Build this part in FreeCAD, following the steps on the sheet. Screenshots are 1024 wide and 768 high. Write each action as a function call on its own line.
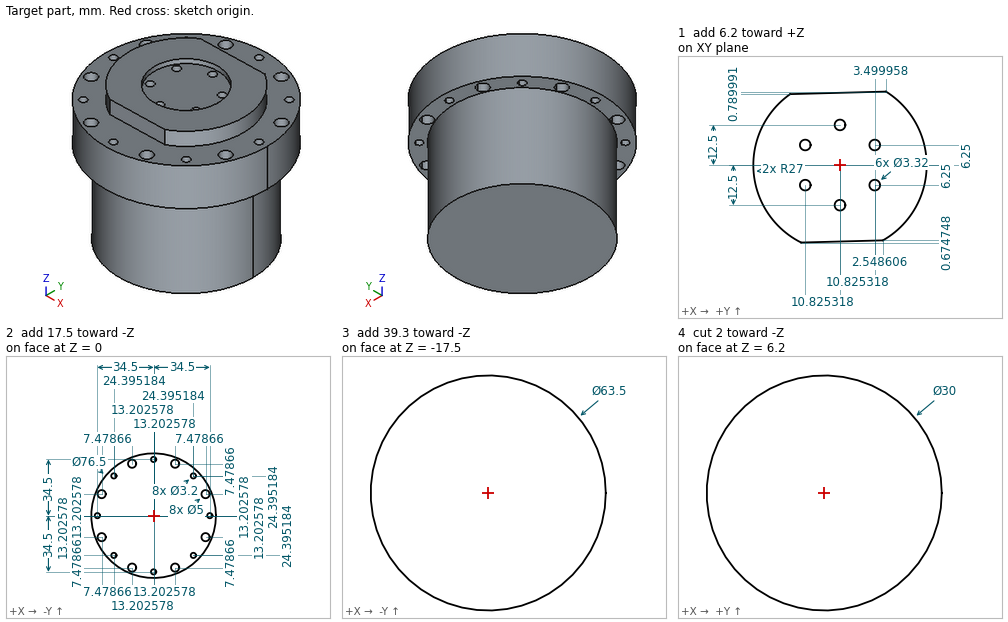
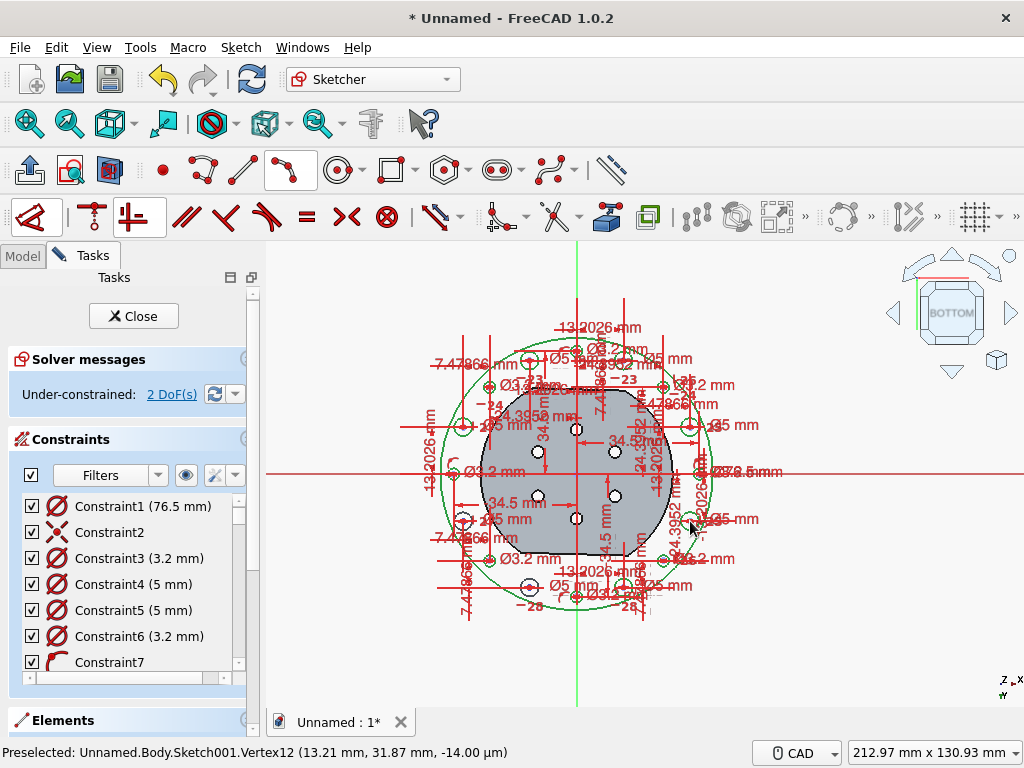
click(463, 521)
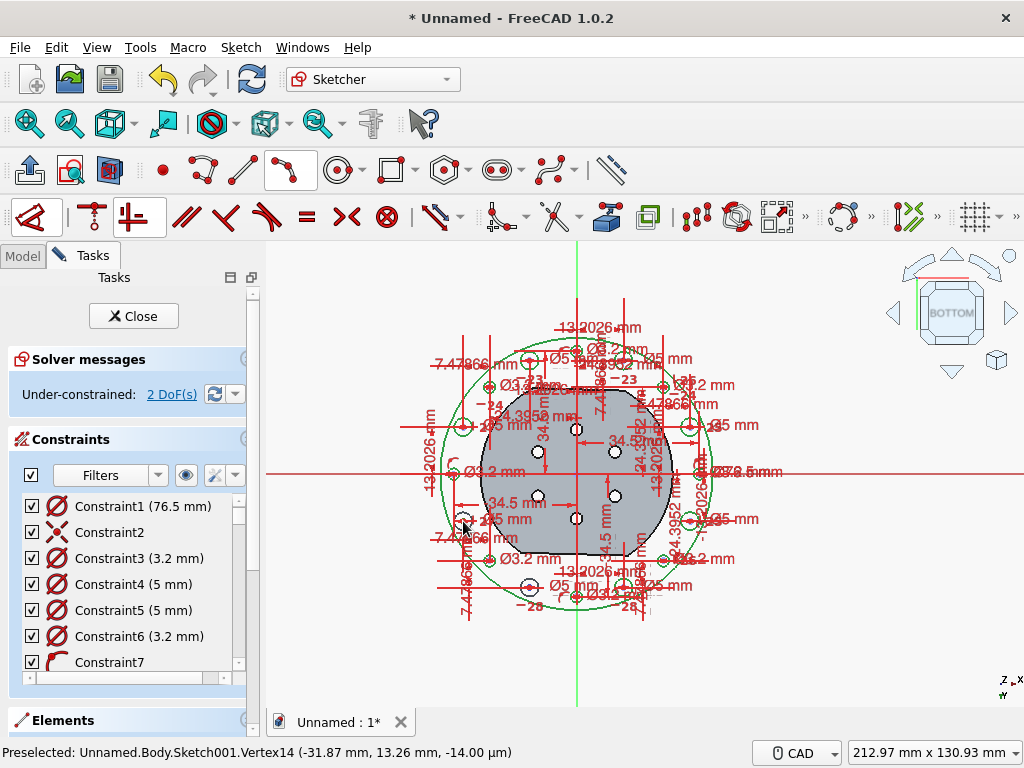
click(56, 218)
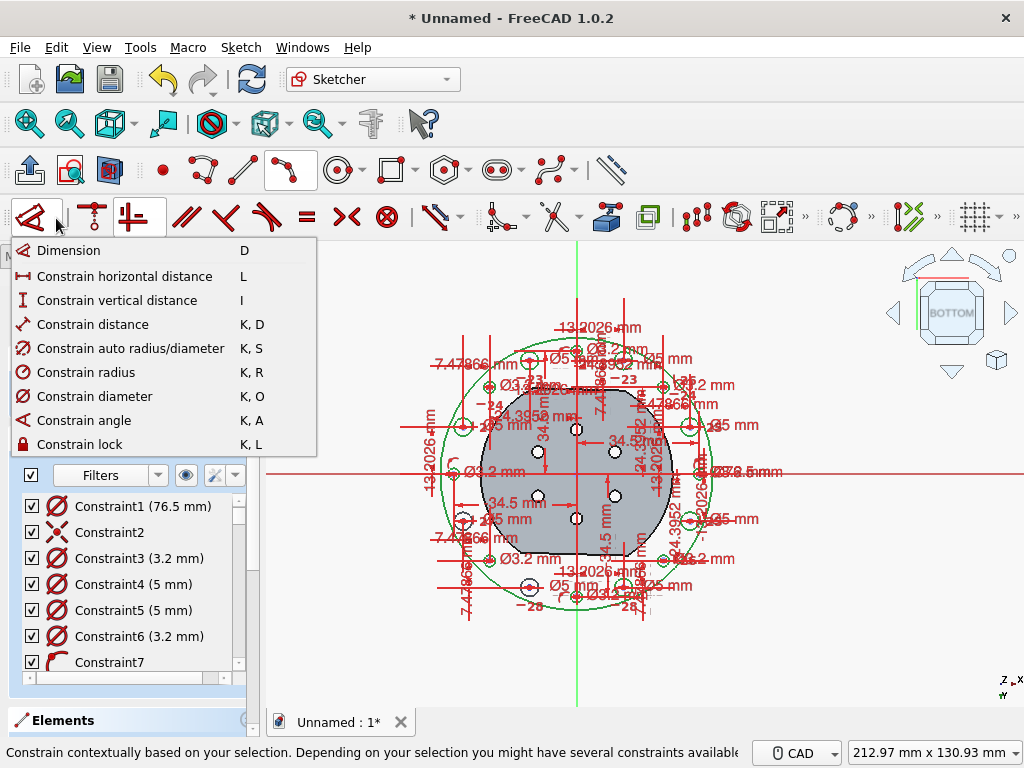
click(164, 300)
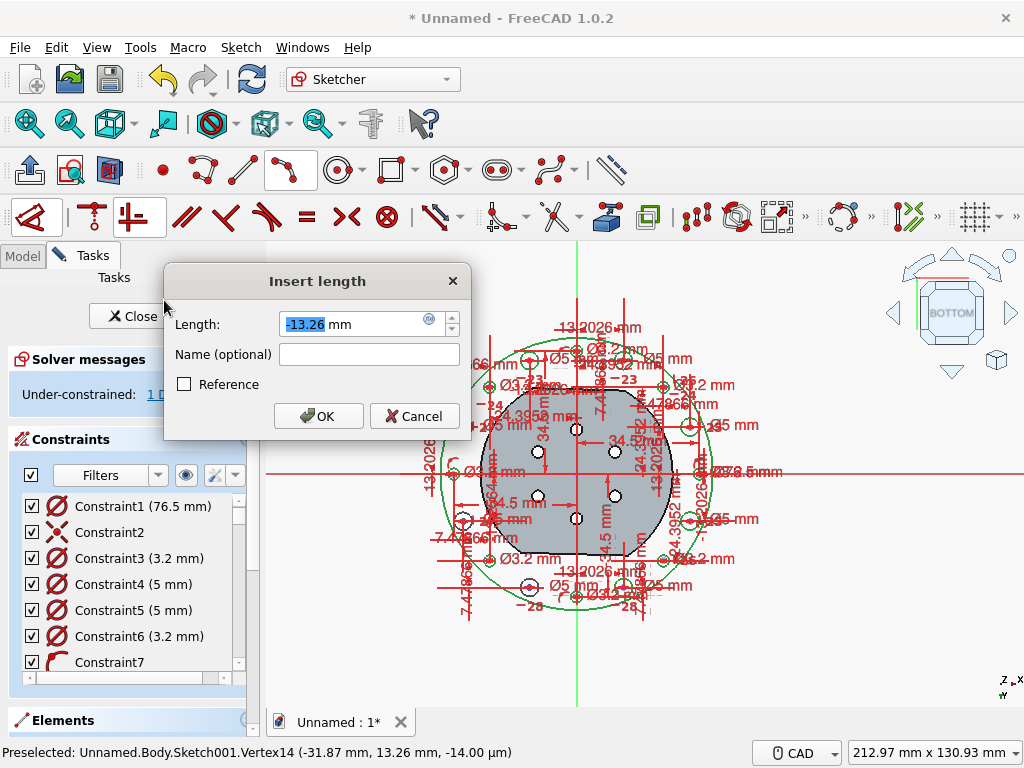
text(-13.202578)
key(Return)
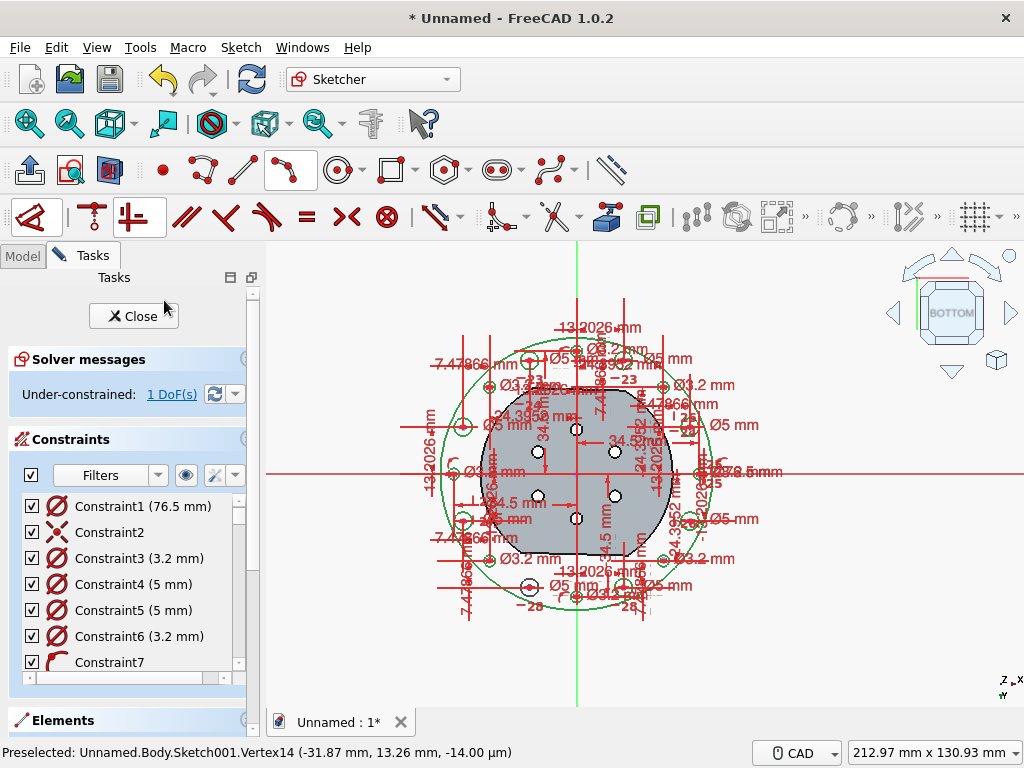
click(530, 588)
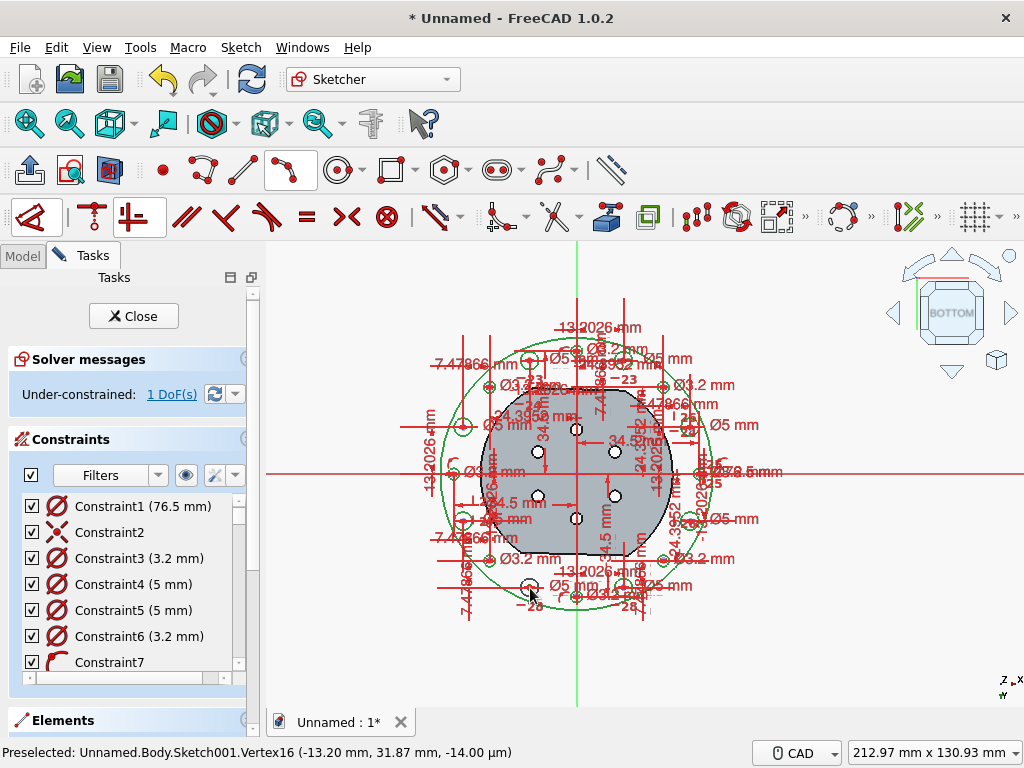
click(56, 218)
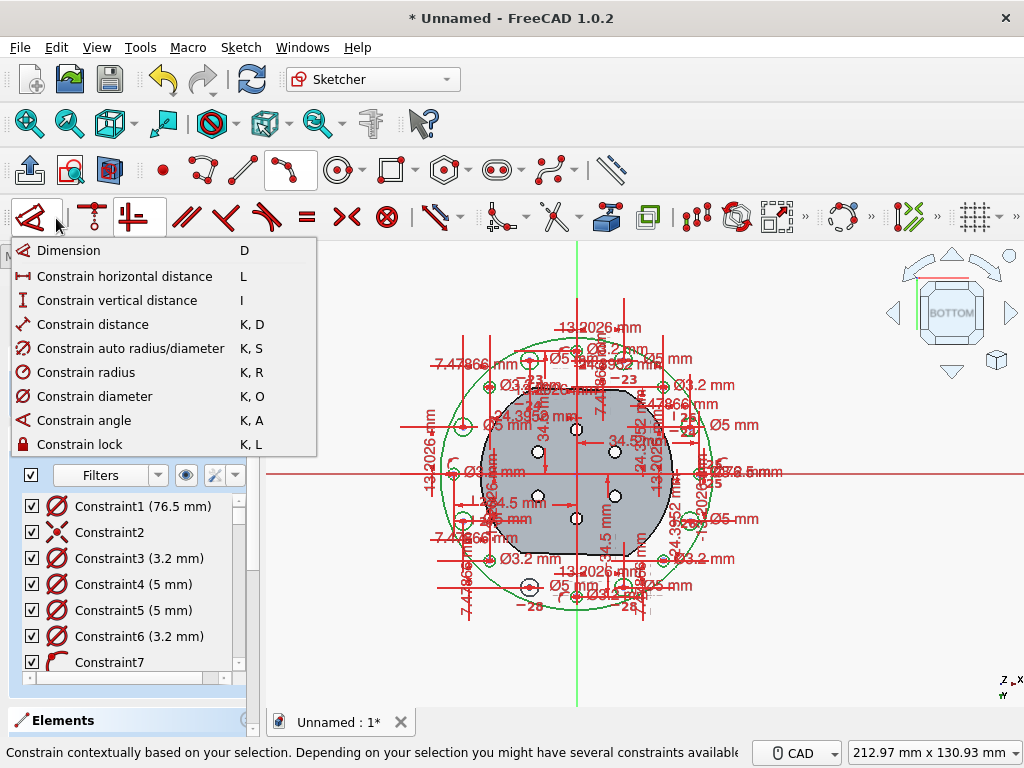
click(164, 276)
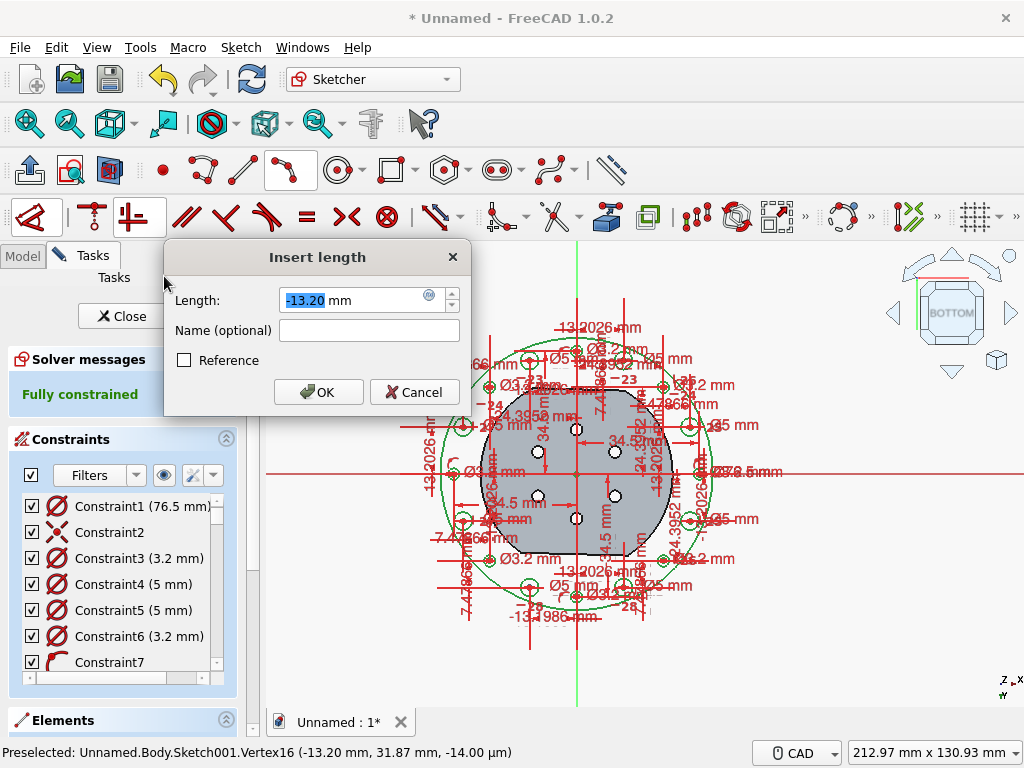
text(-13.202578)
key(Return)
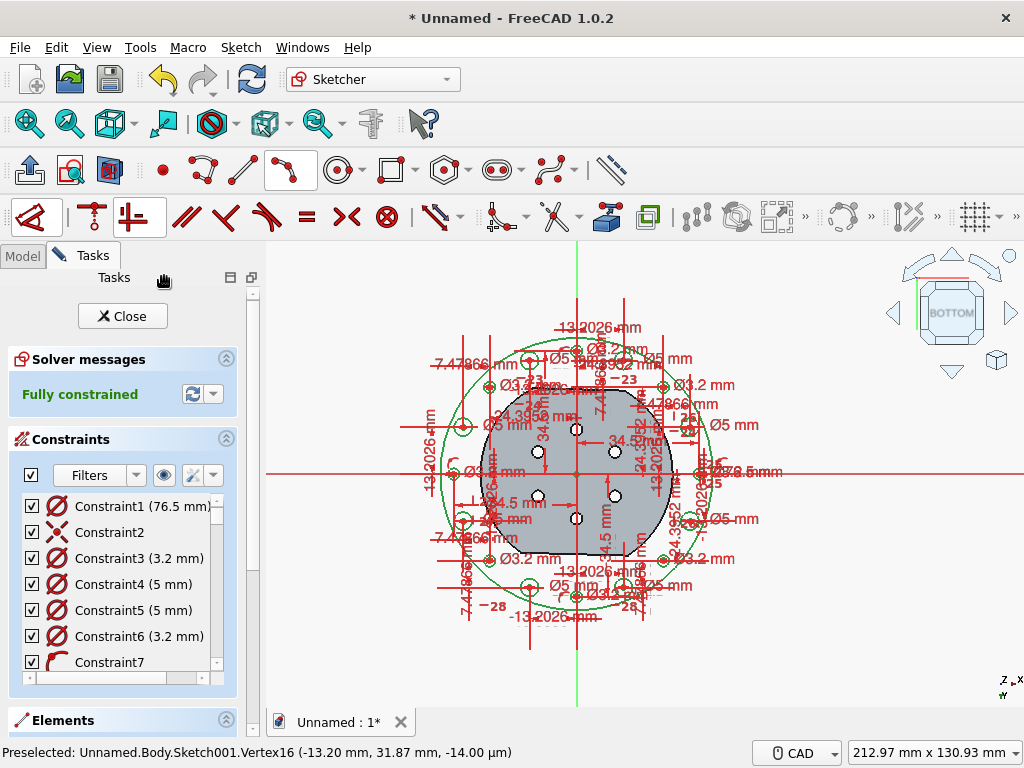
click(123, 316)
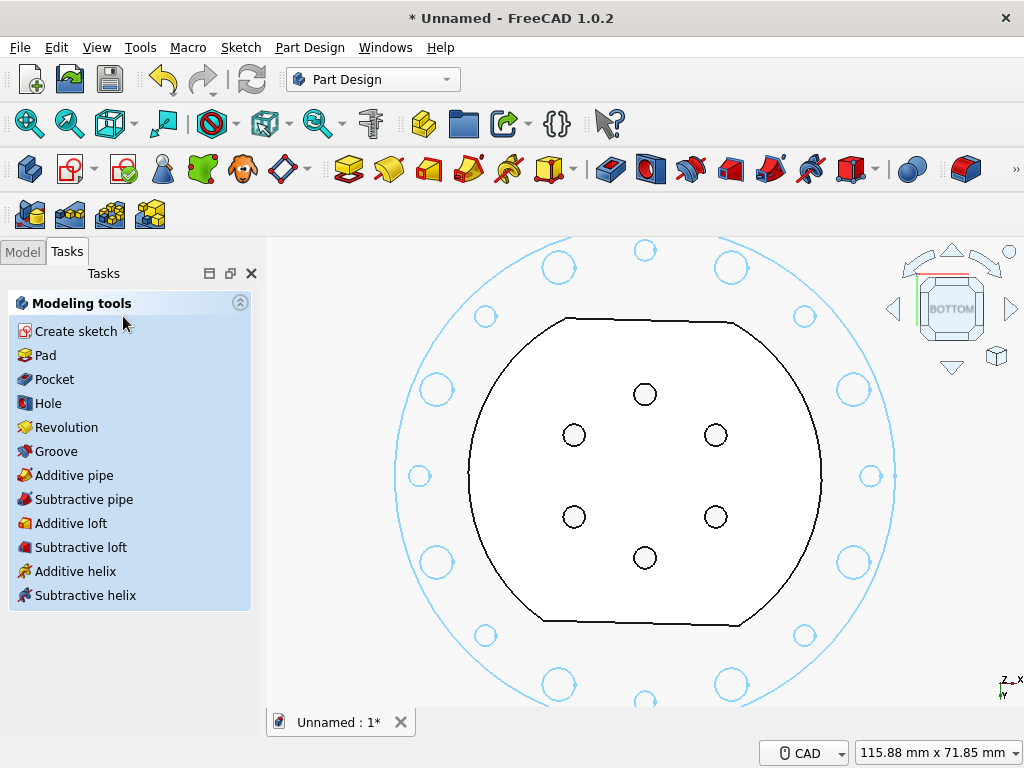
click(350, 170)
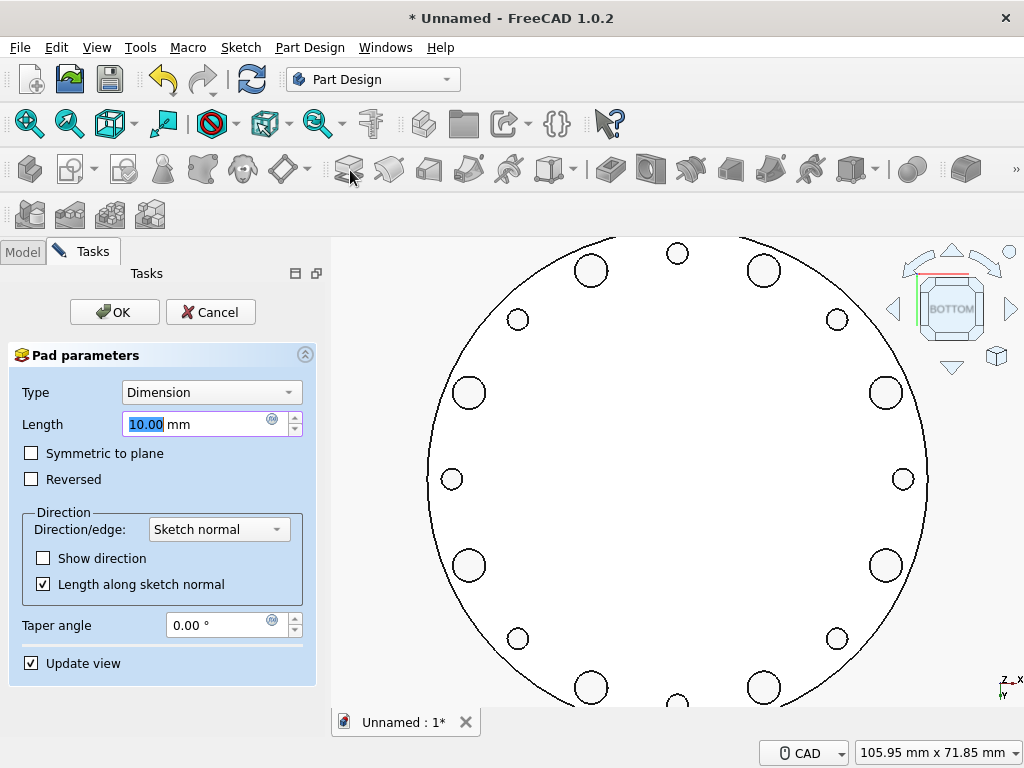
text(17.5)
key(Tab)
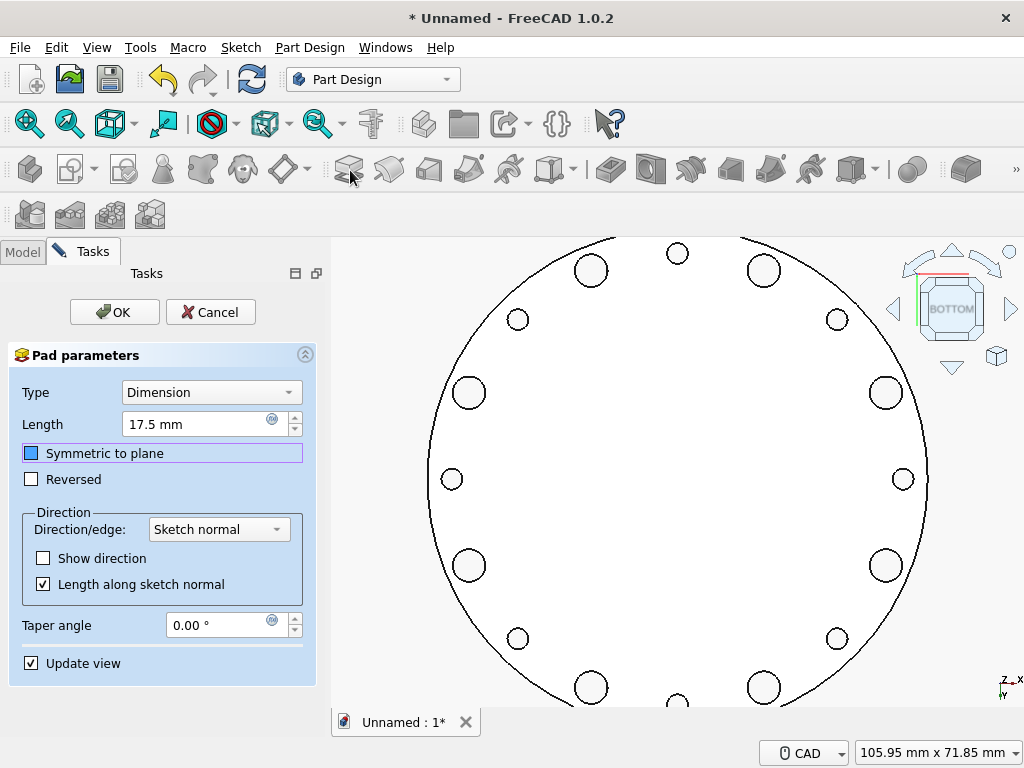
click(115, 312)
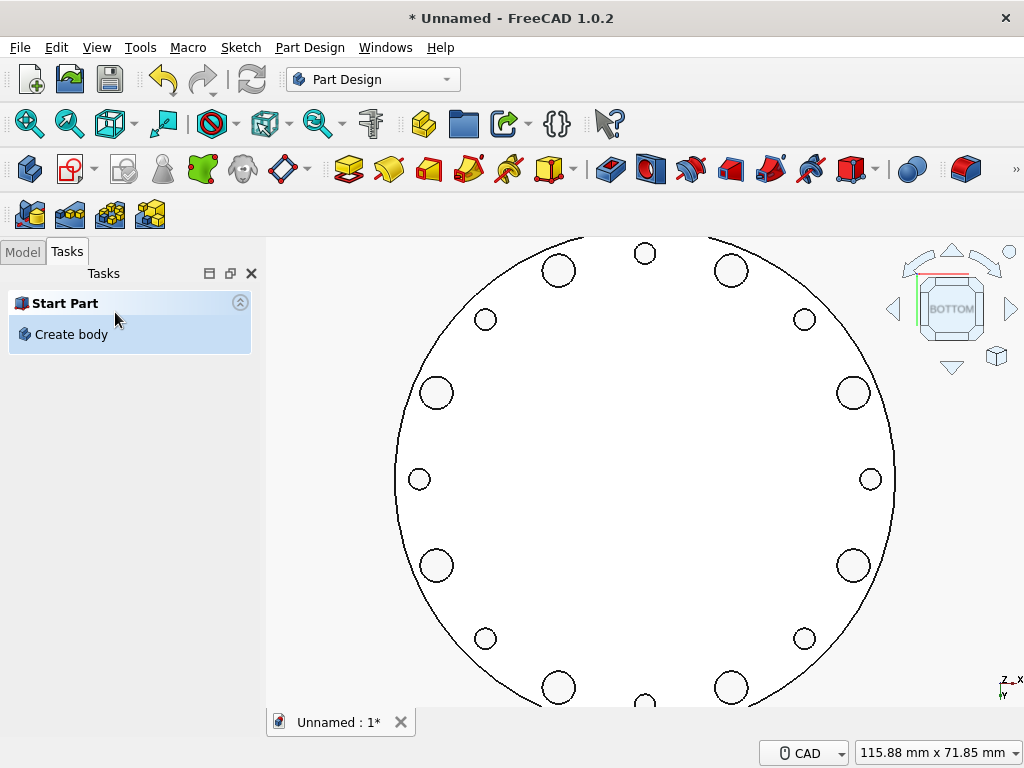
click(30, 124)